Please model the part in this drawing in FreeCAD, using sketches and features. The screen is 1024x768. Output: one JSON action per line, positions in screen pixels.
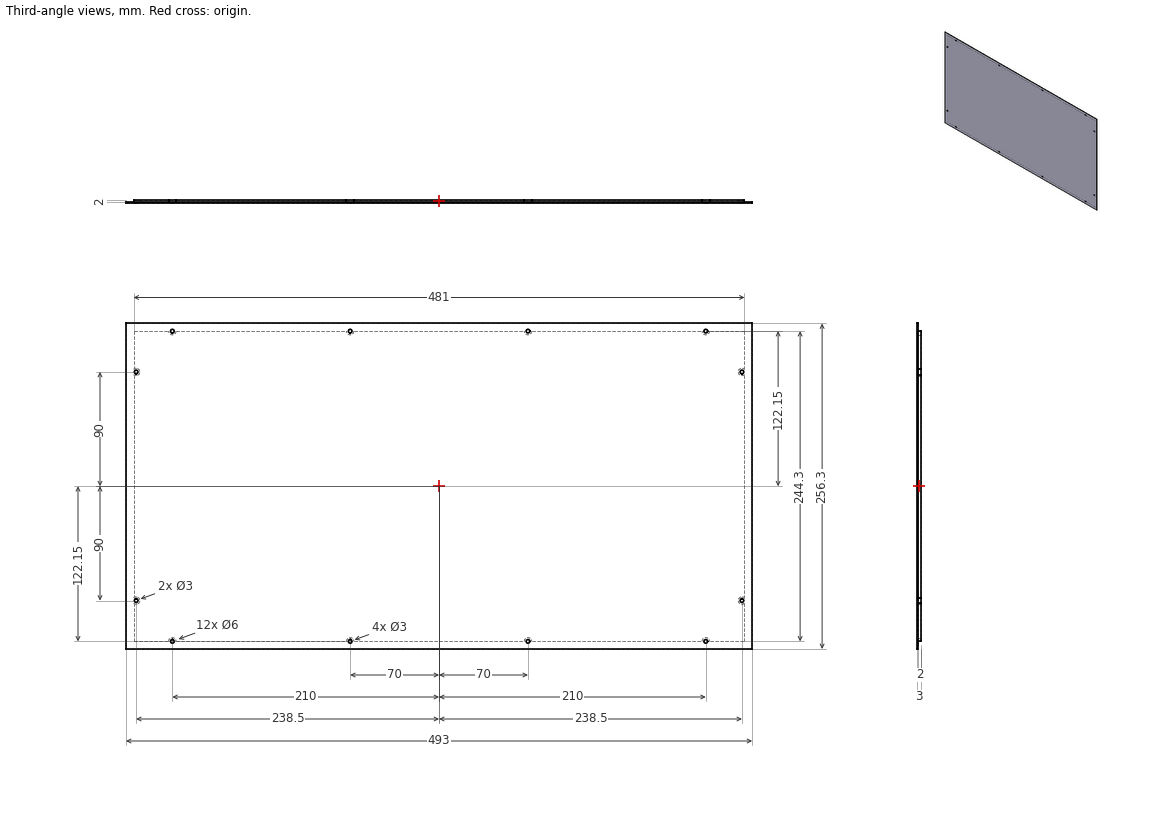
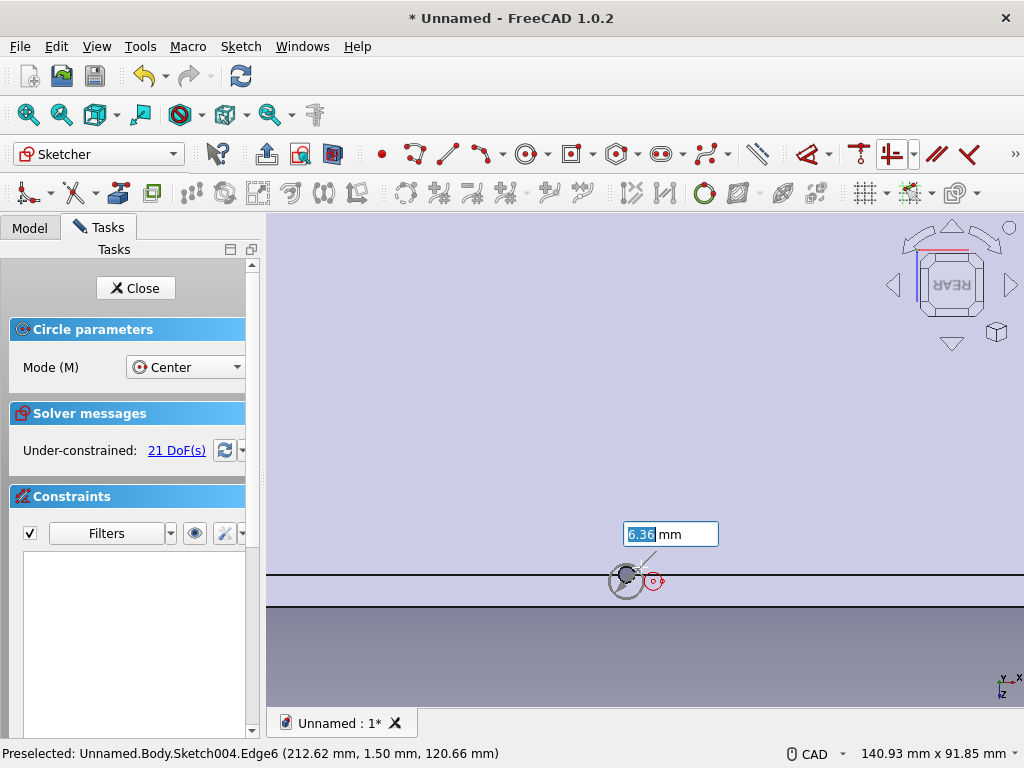
{"action": "left_click", "coordinate": [638, 563]}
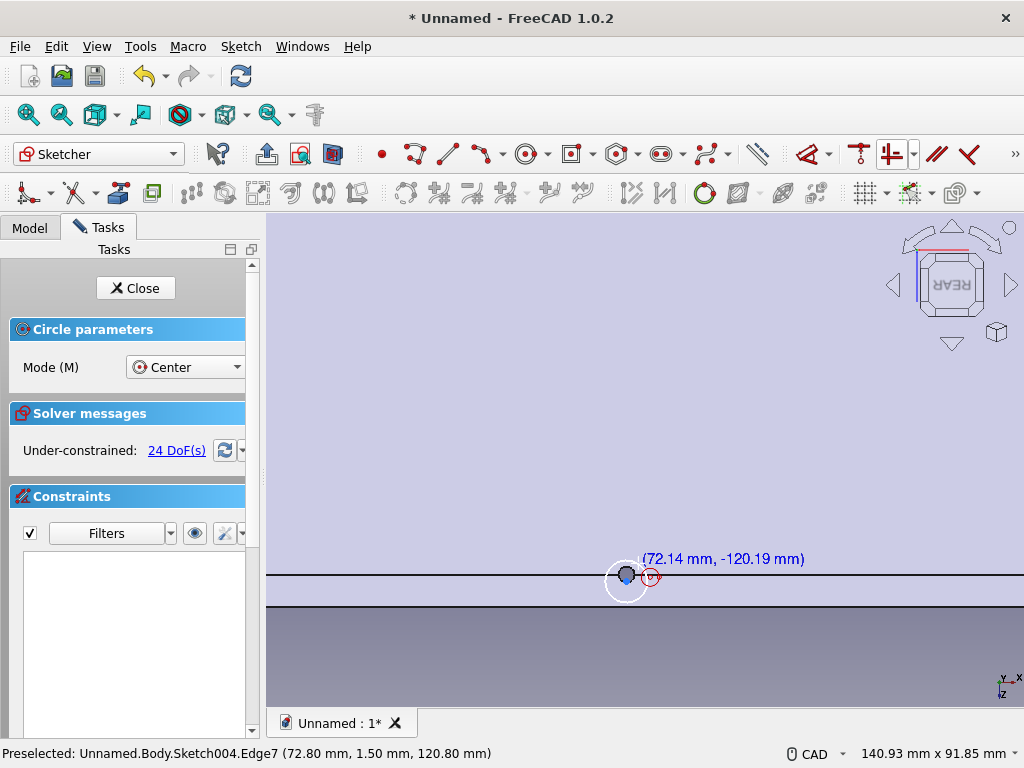
{"action": "scroll", "coordinate": [641, 567], "scroll_direction": "down", "scroll_amount": 9}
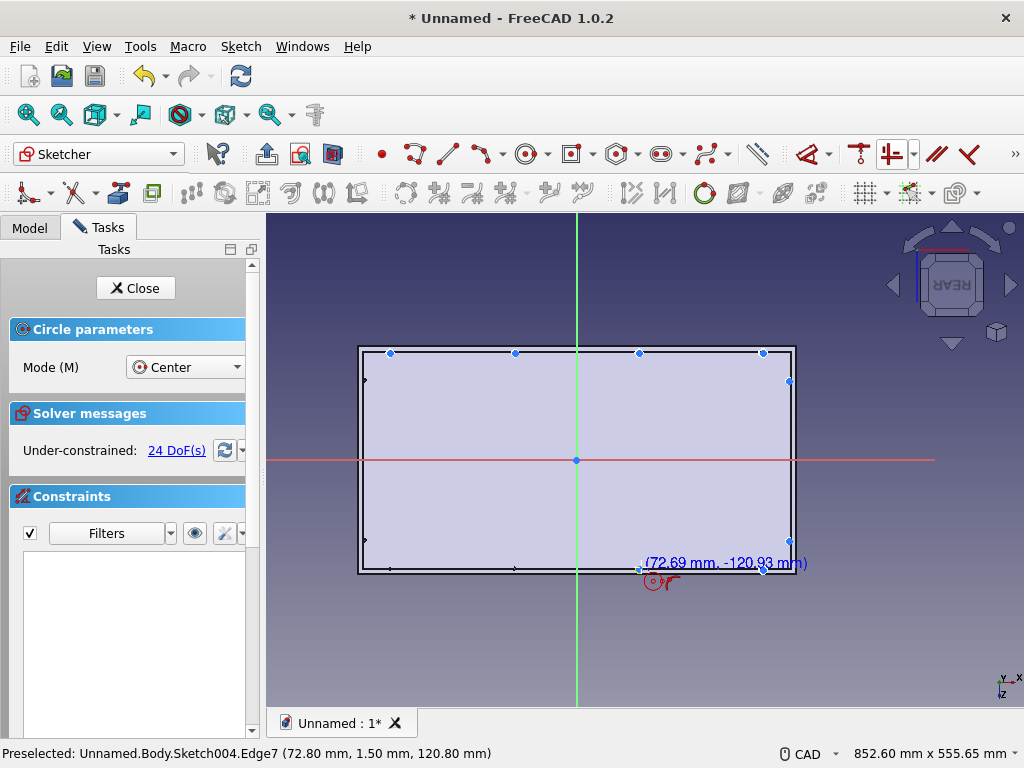
{"action": "scroll", "coordinate": [515, 569], "scroll_direction": "up", "scroll_amount": 11}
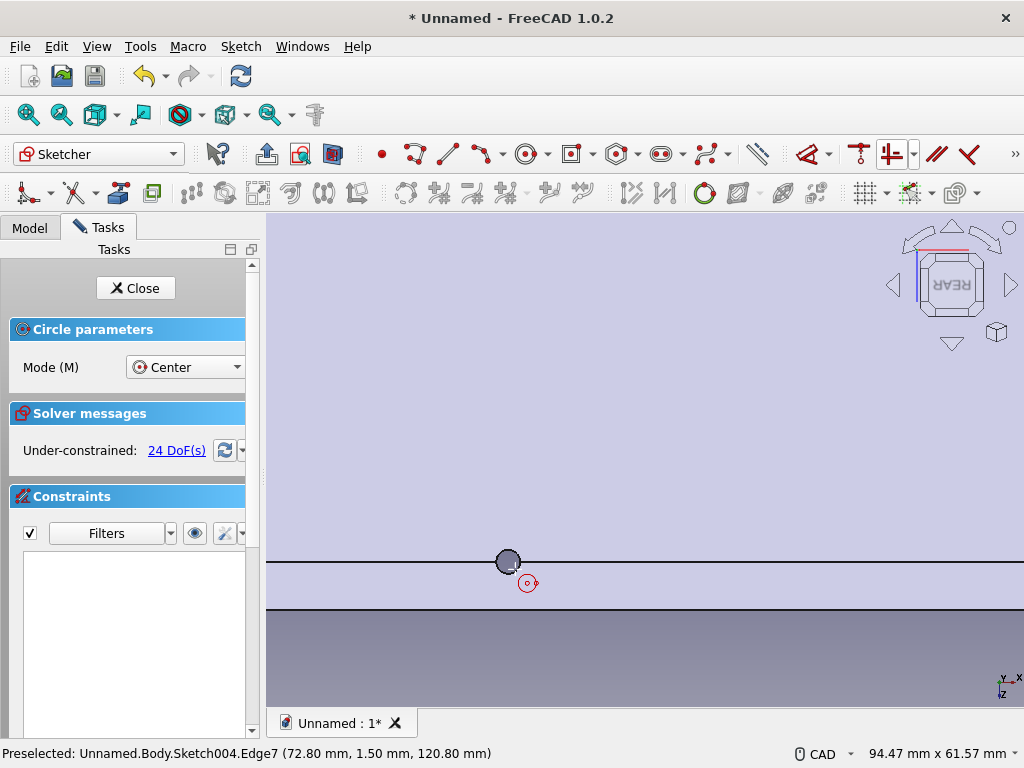
{"action": "scroll", "coordinate": [515, 569], "scroll_direction": "down", "scroll_amount": 11}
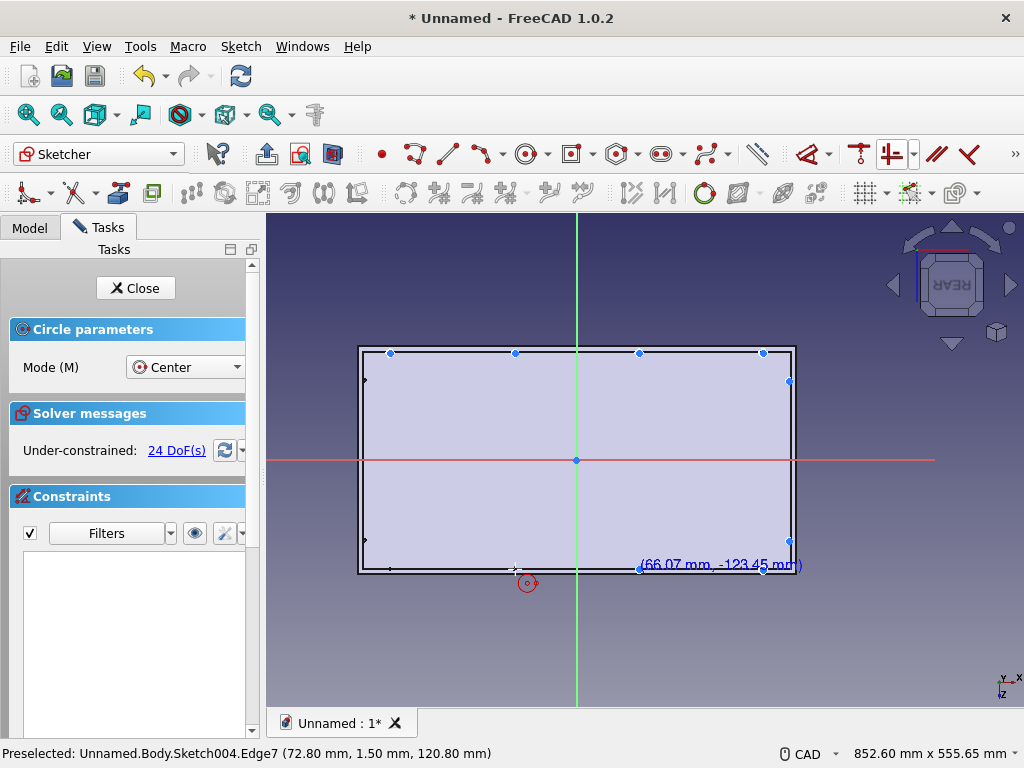
{"action": "left_click", "coordinate": [515, 569]}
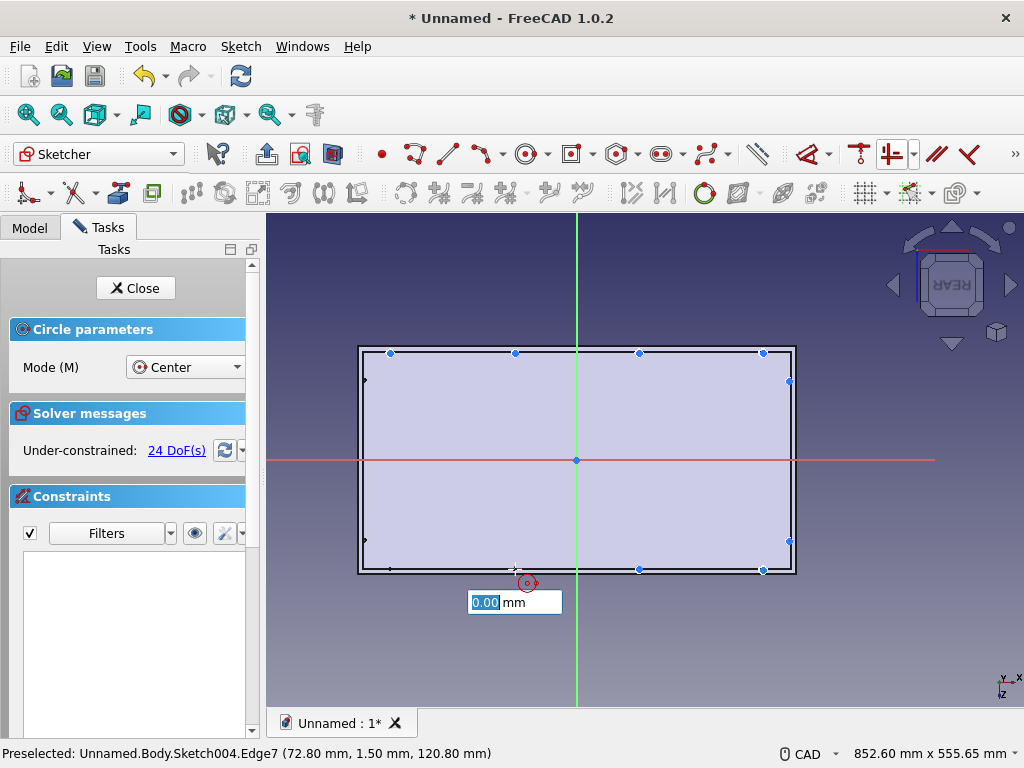
{"action": "scroll", "coordinate": [516, 567], "scroll_direction": "up", "scroll_amount": 9}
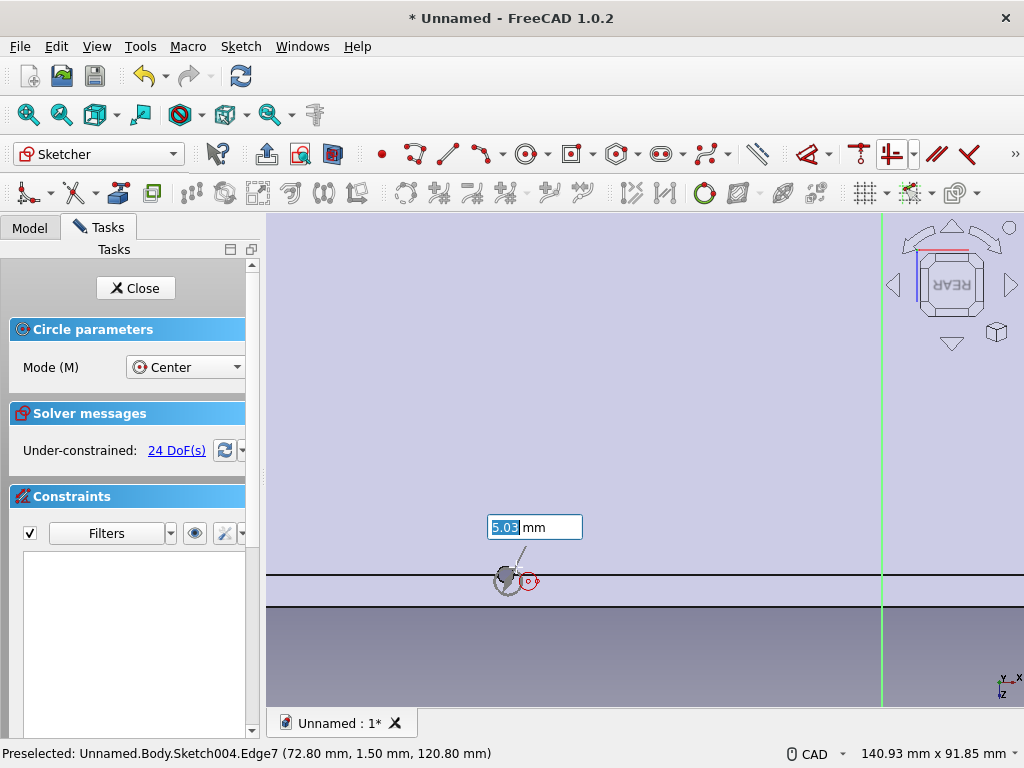
{"action": "left_click", "coordinate": [517, 563]}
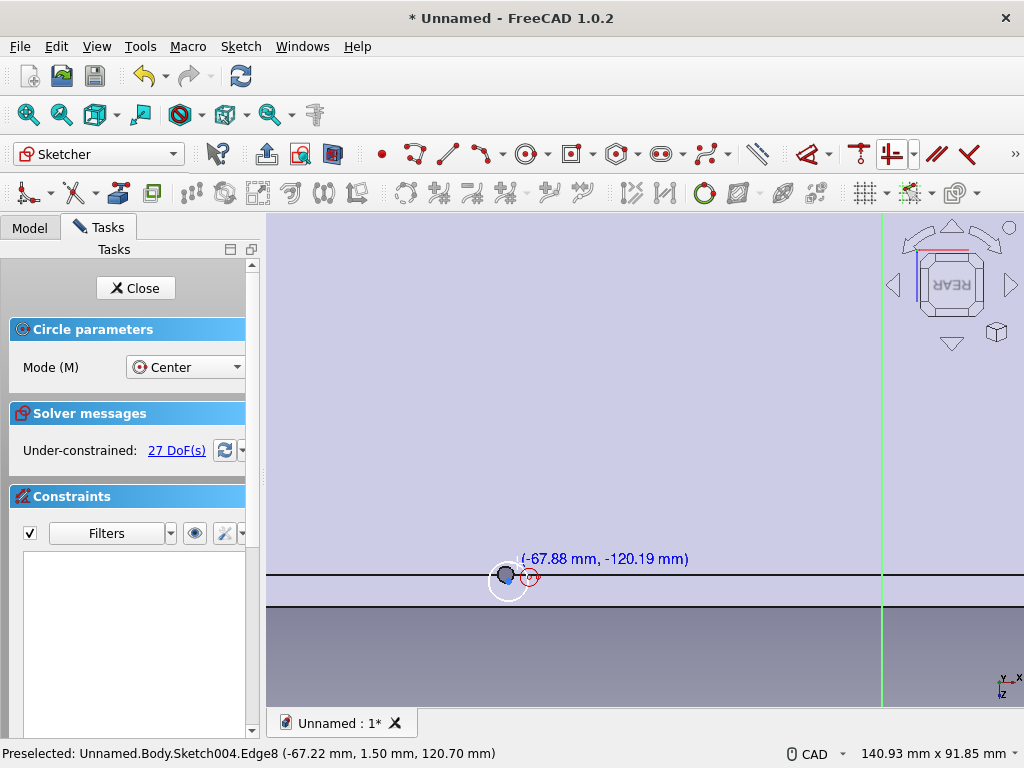
{"action": "scroll", "coordinate": [516, 567], "scroll_direction": "down", "scroll_amount": 9}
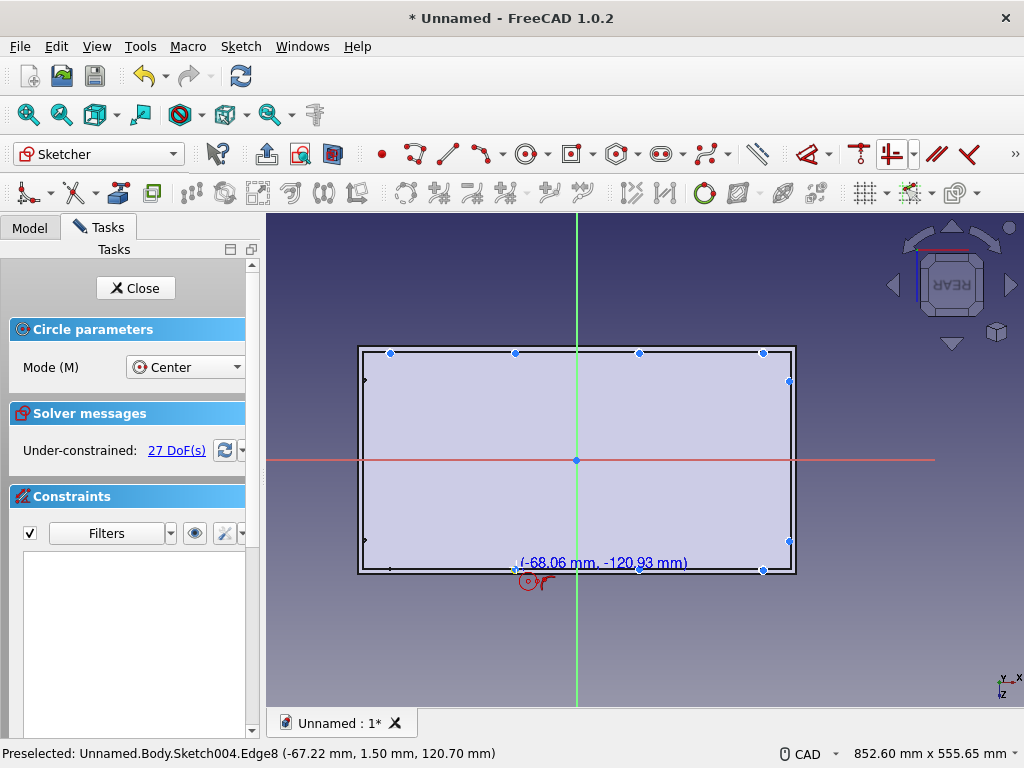
{"action": "scroll", "coordinate": [390, 569], "scroll_direction": "up", "scroll_amount": 11}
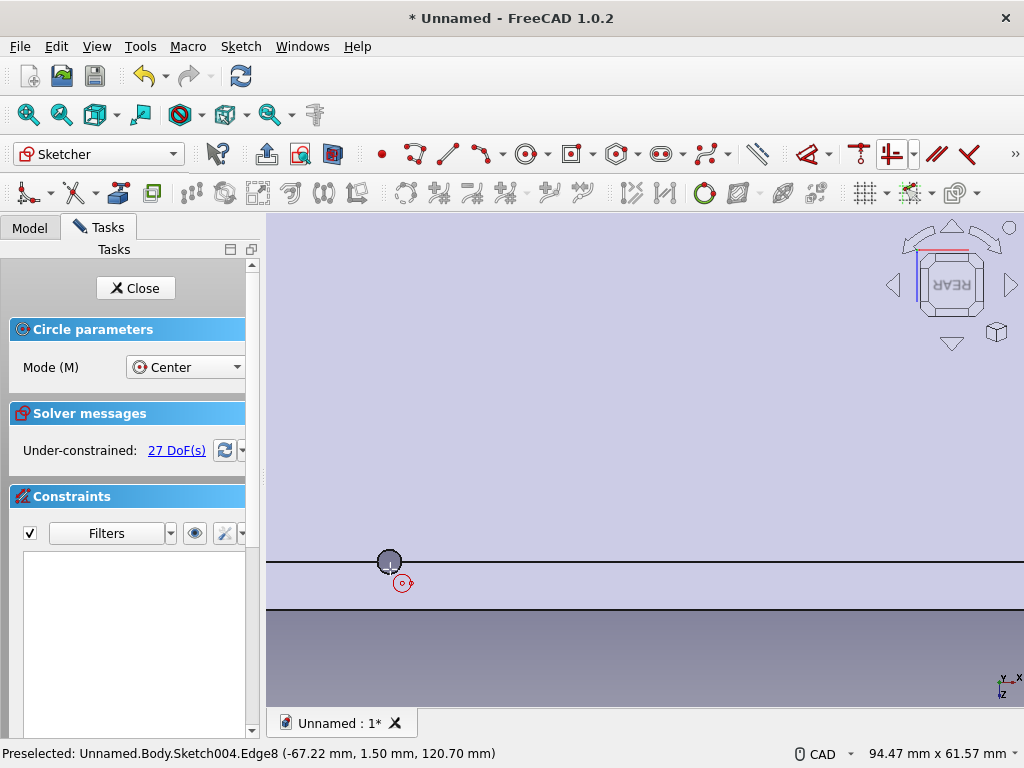
{"action": "scroll", "coordinate": [390, 569], "scroll_direction": "down", "scroll_amount": 11}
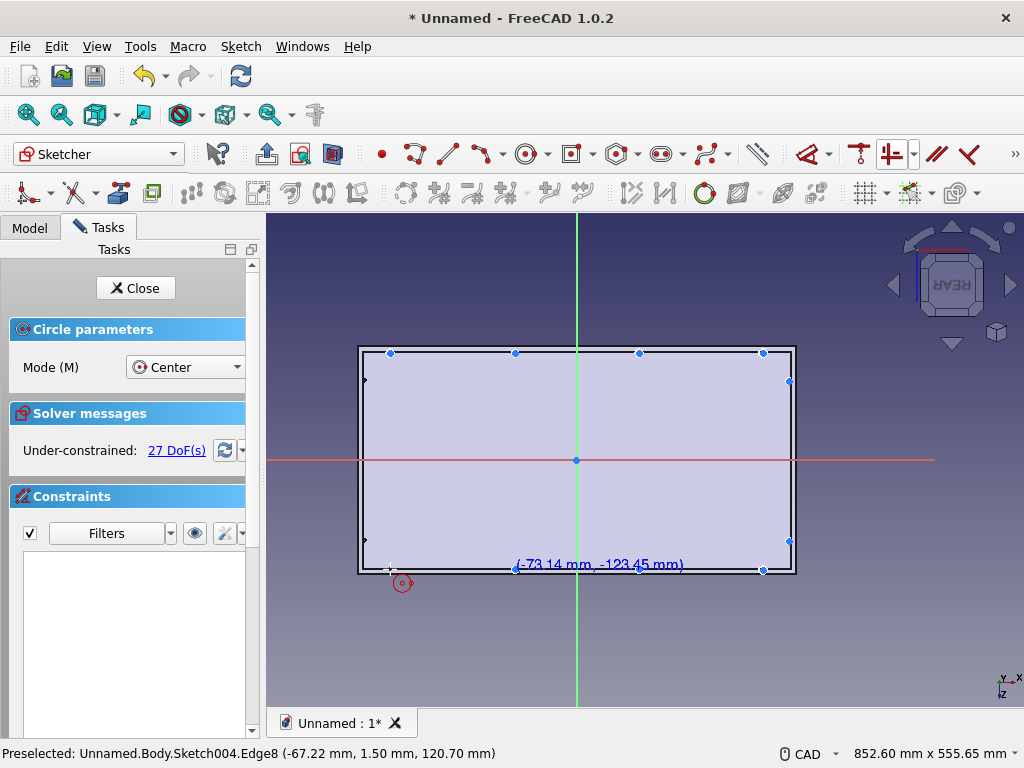
{"action": "left_click", "coordinate": [390, 569]}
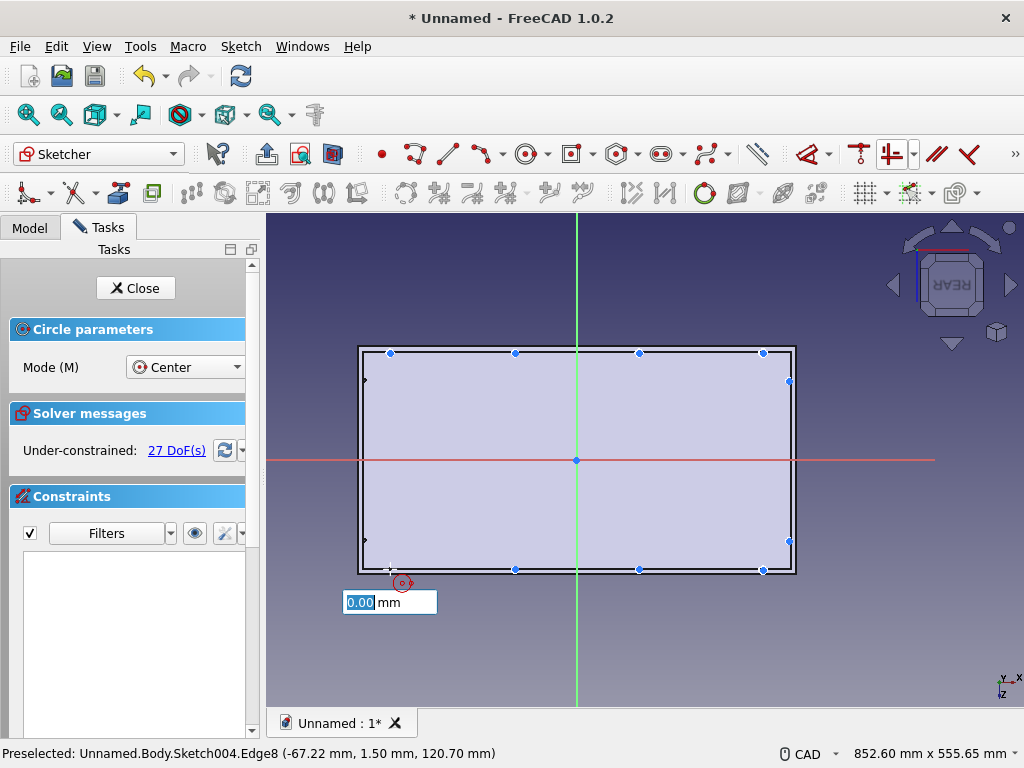
{"action": "scroll", "coordinate": [392, 567], "scroll_direction": "up", "scroll_amount": 9}